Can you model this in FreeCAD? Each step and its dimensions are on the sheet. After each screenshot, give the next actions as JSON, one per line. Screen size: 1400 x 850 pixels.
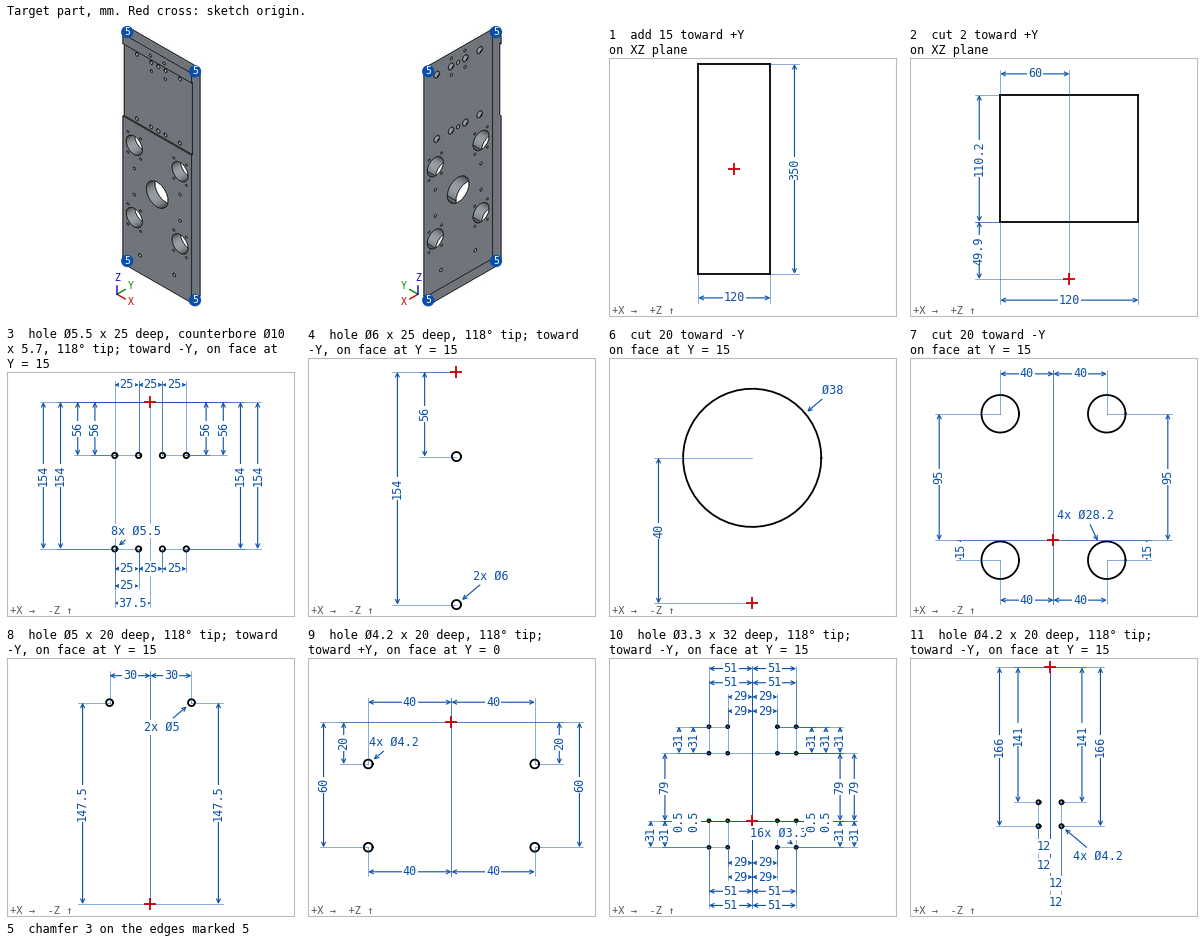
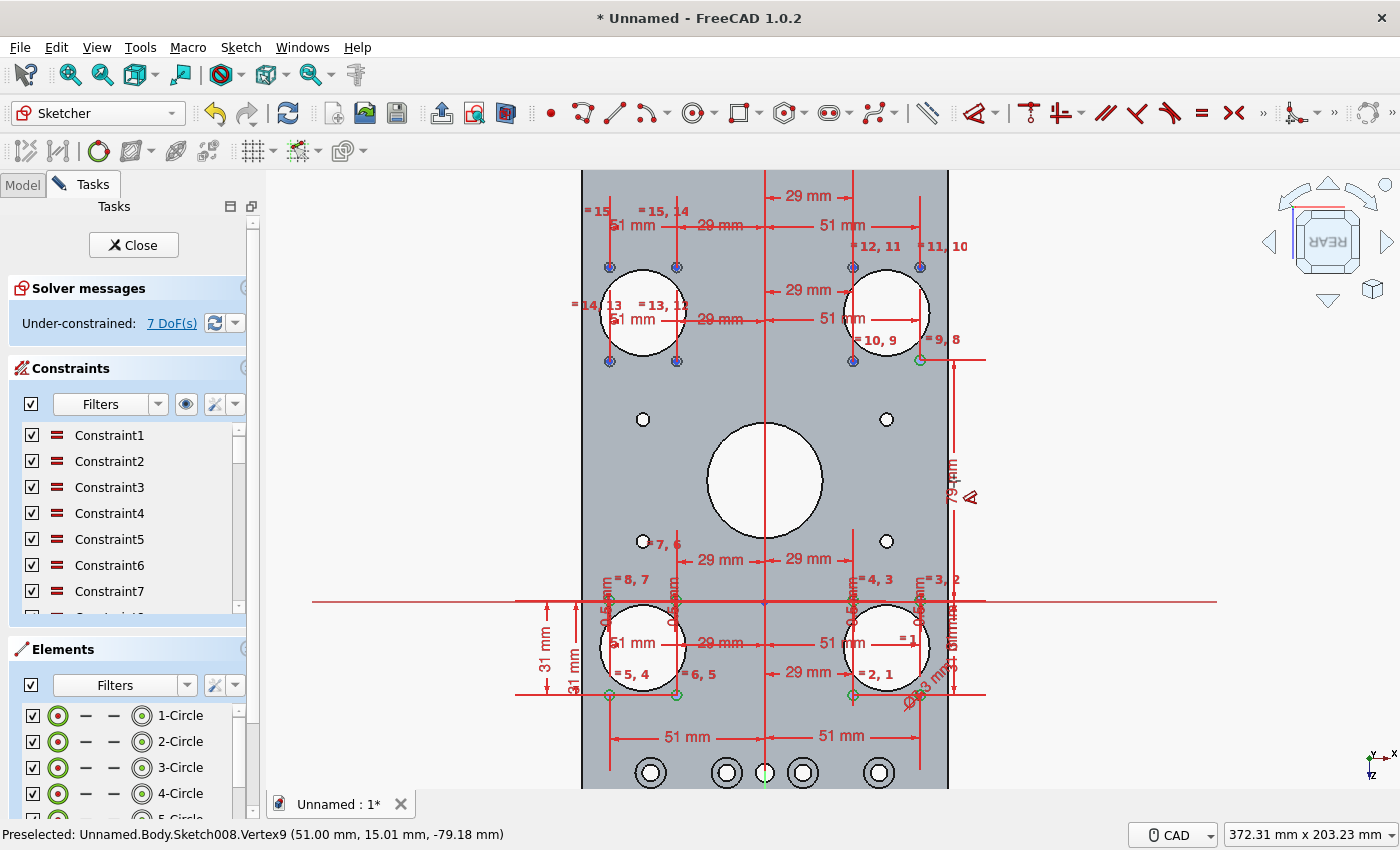
{"action": "left_click", "coordinate": [853, 601]}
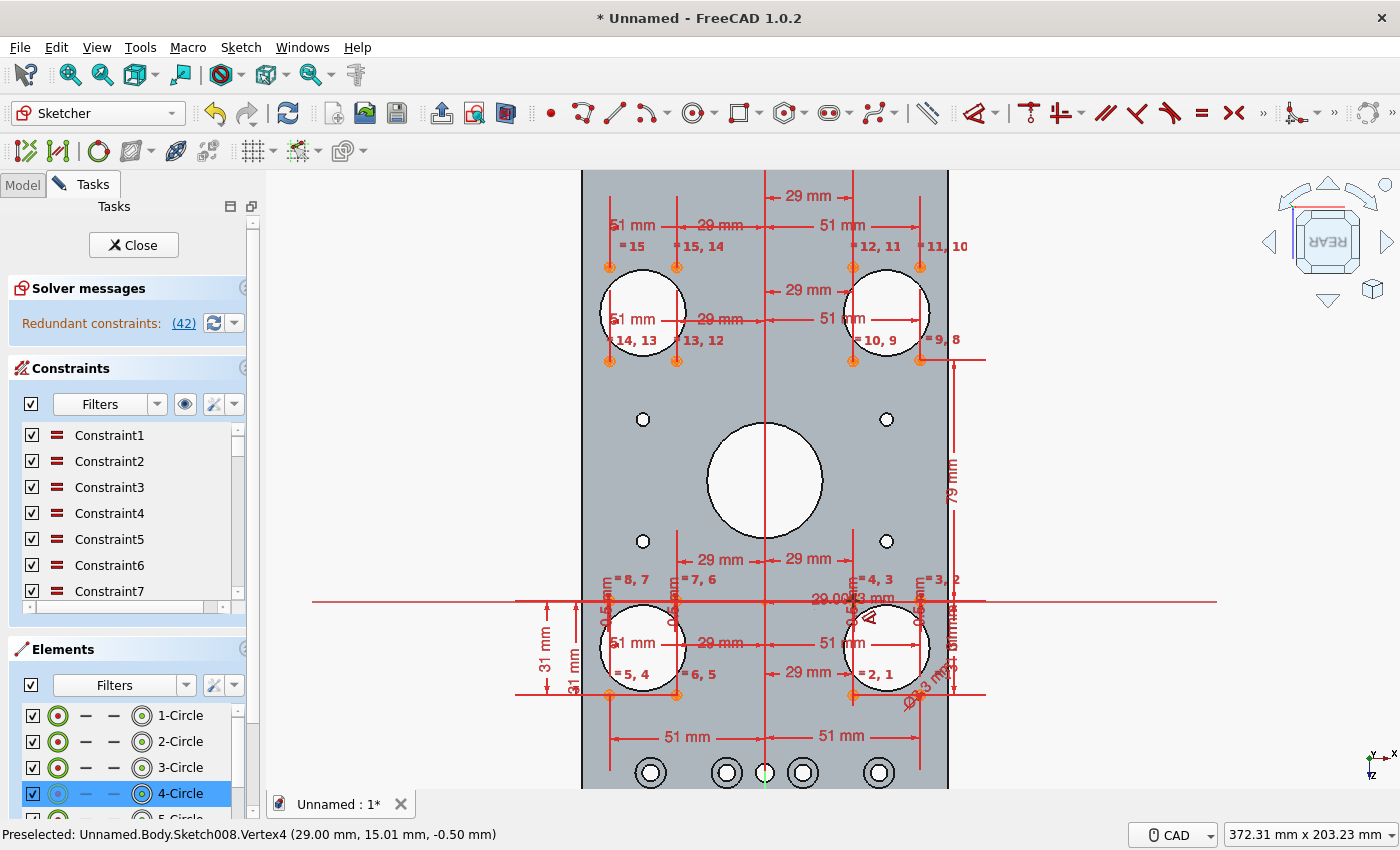
{"action": "left_click", "coordinate": [853, 361]}
{"action": "left_click", "coordinate": [887, 426]}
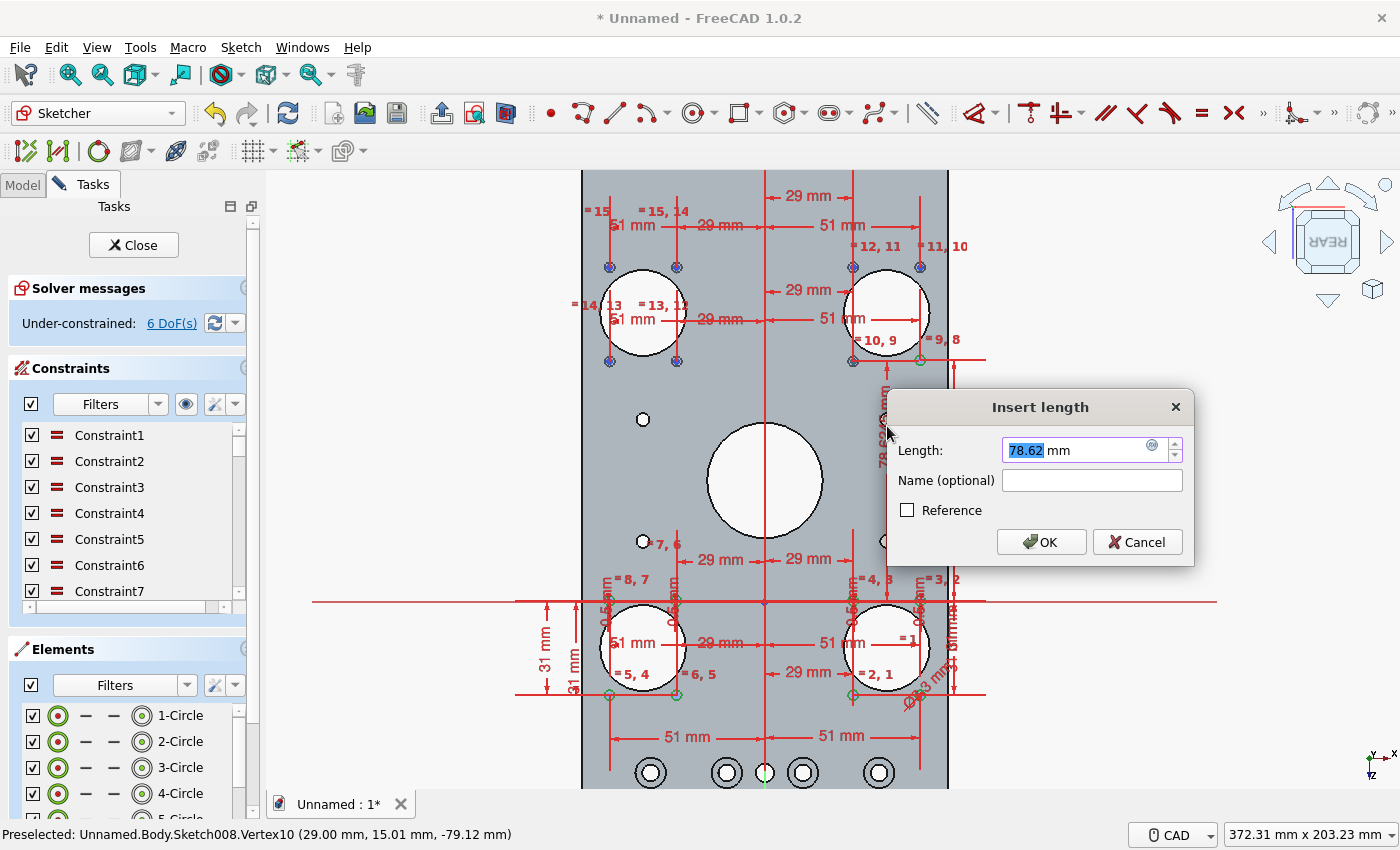
{"action": "type", "text": "79"}
{"action": "key", "text": "Return"}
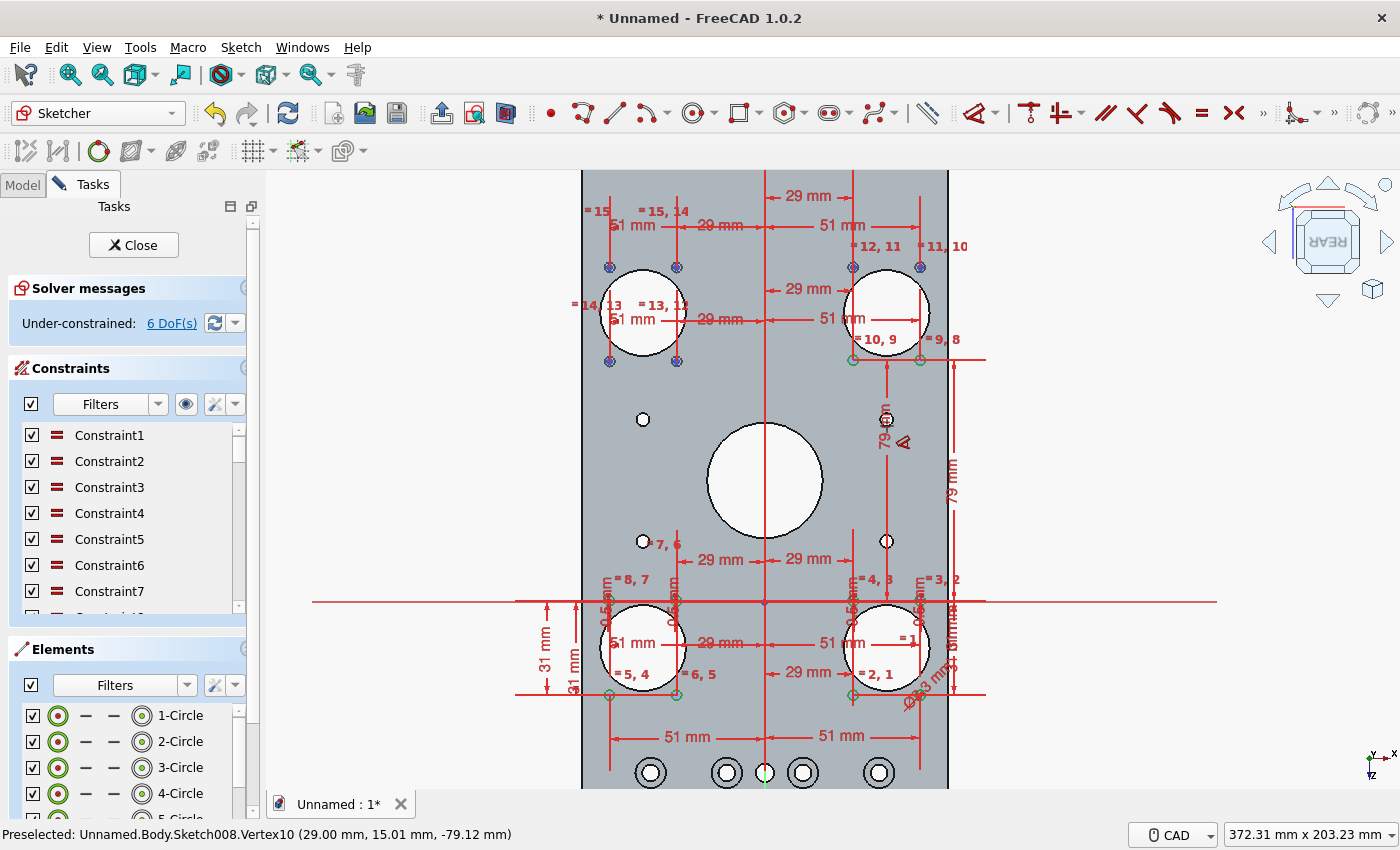
{"action": "left_click", "coordinate": [920, 360]}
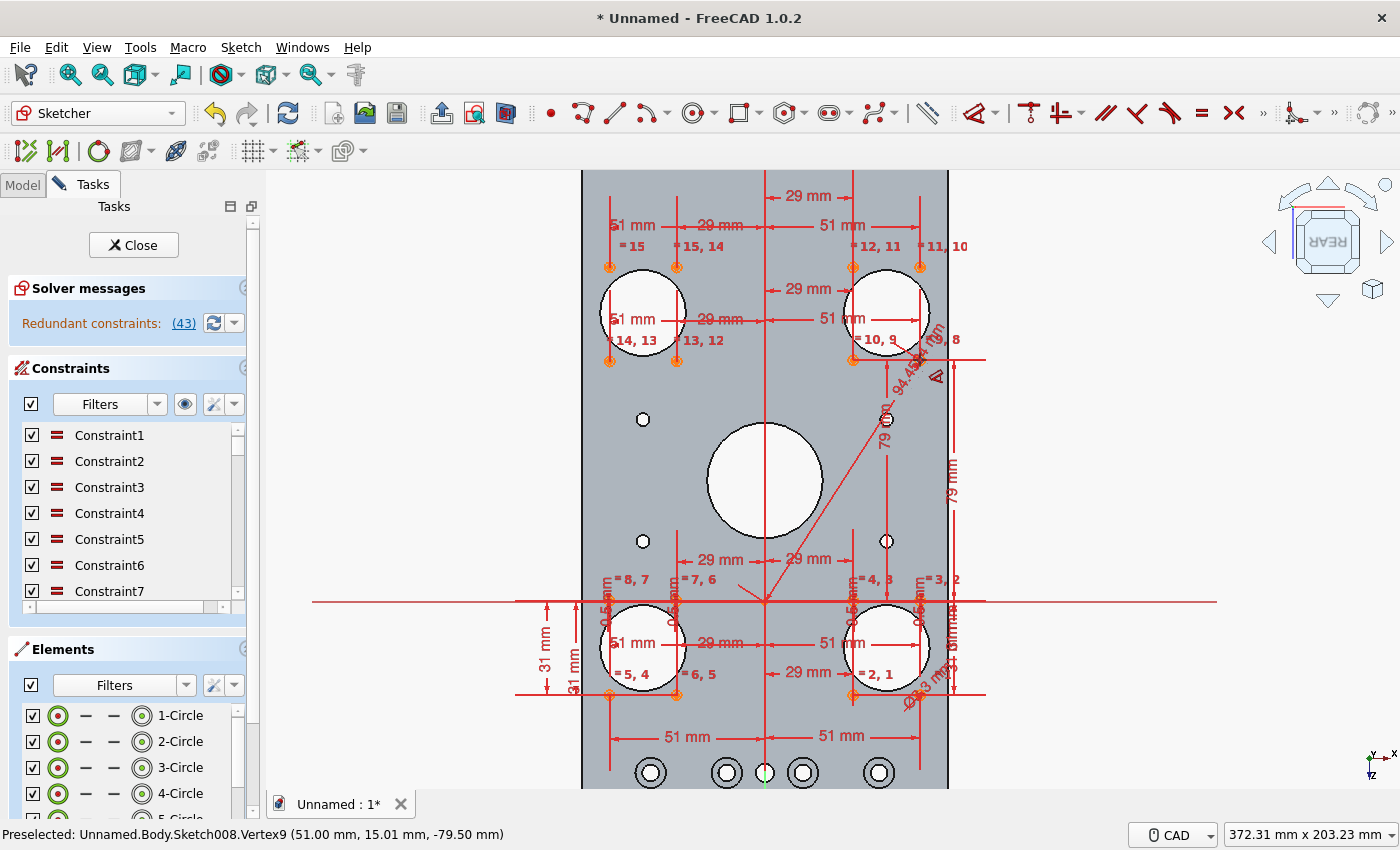
{"action": "left_click", "coordinate": [920, 267]}
{"action": "left_click", "coordinate": [954, 314]}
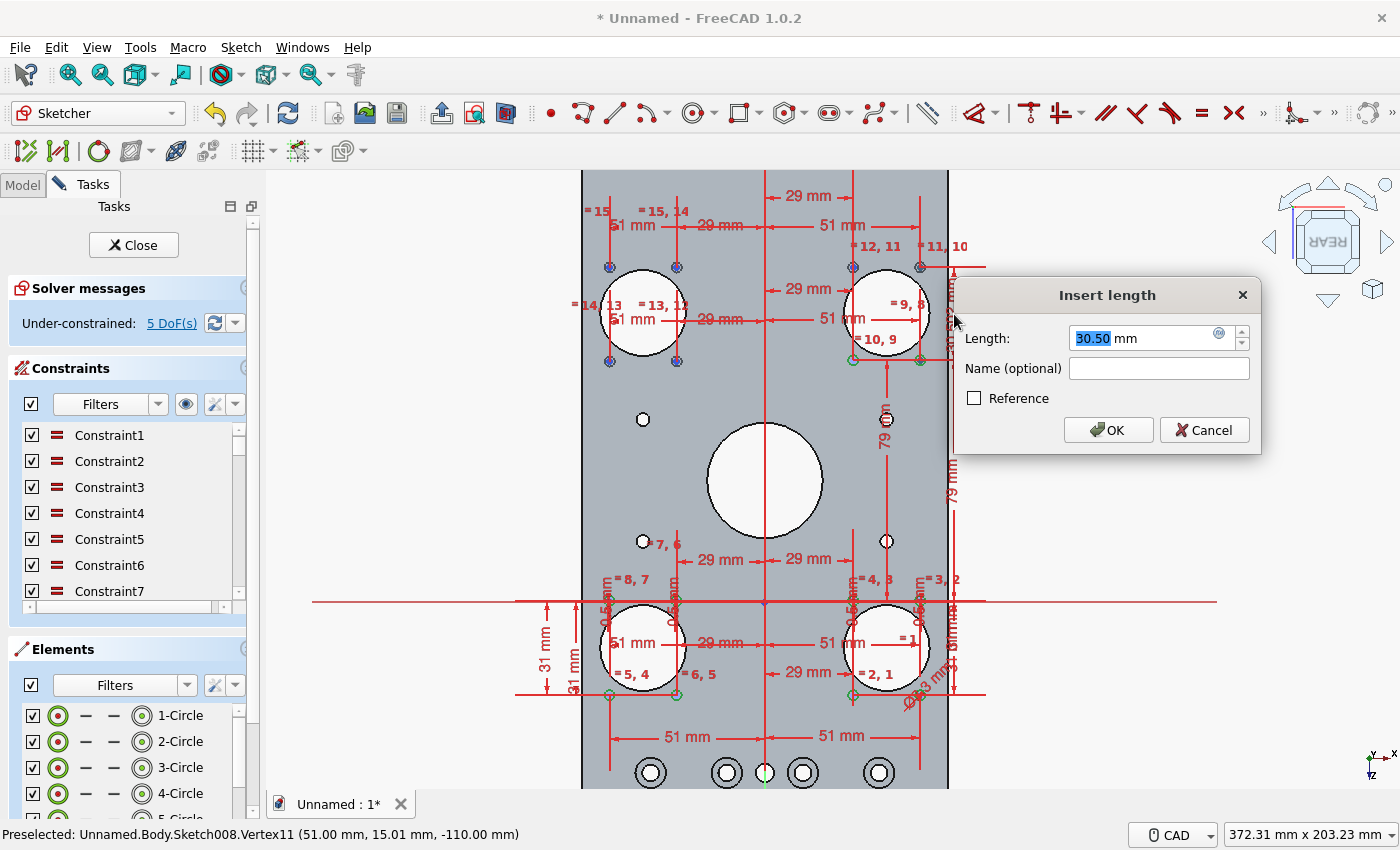
{"action": "type", "text": "31"}
{"action": "key", "text": "Return"}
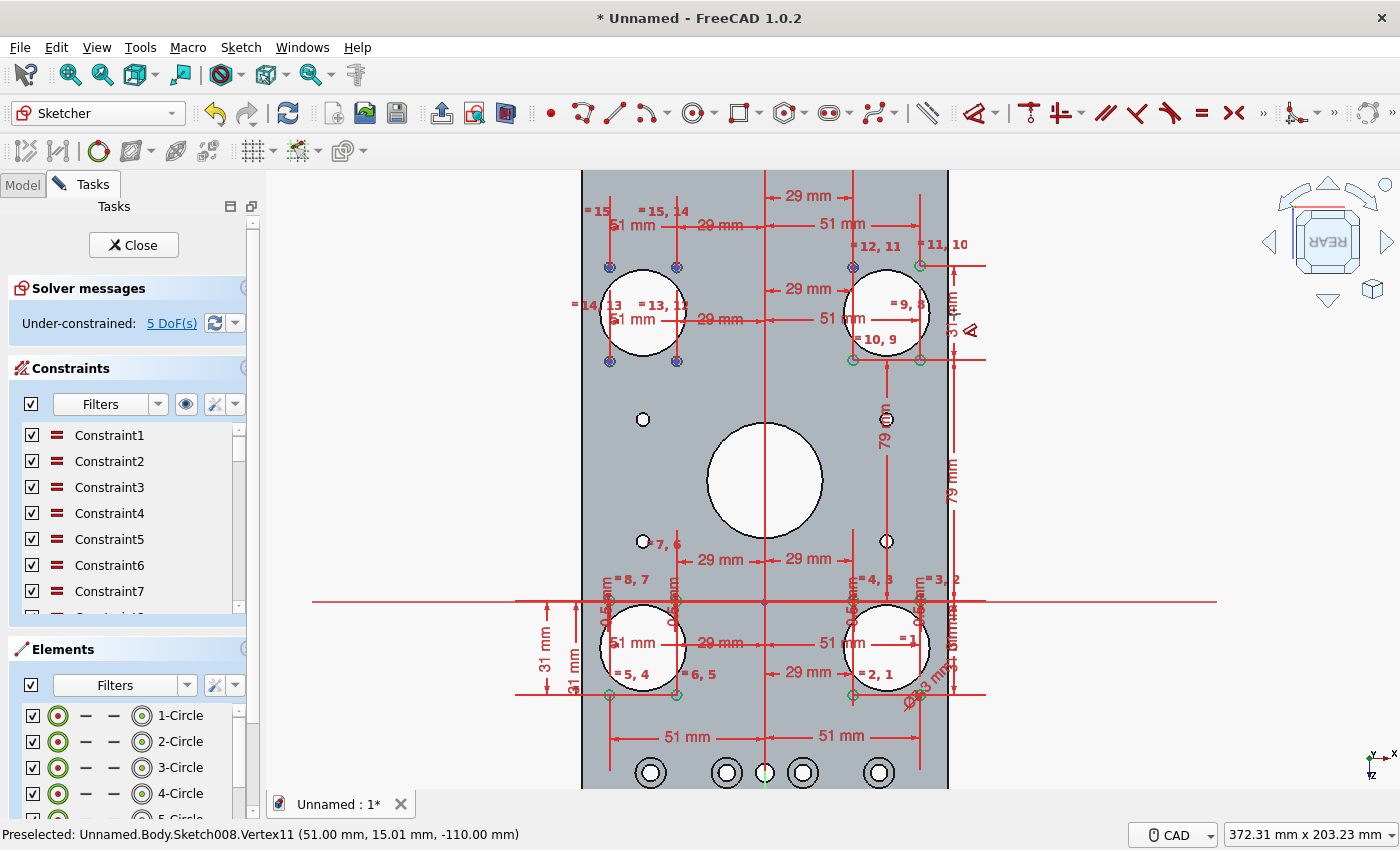
{"action": "left_click", "coordinate": [853, 360]}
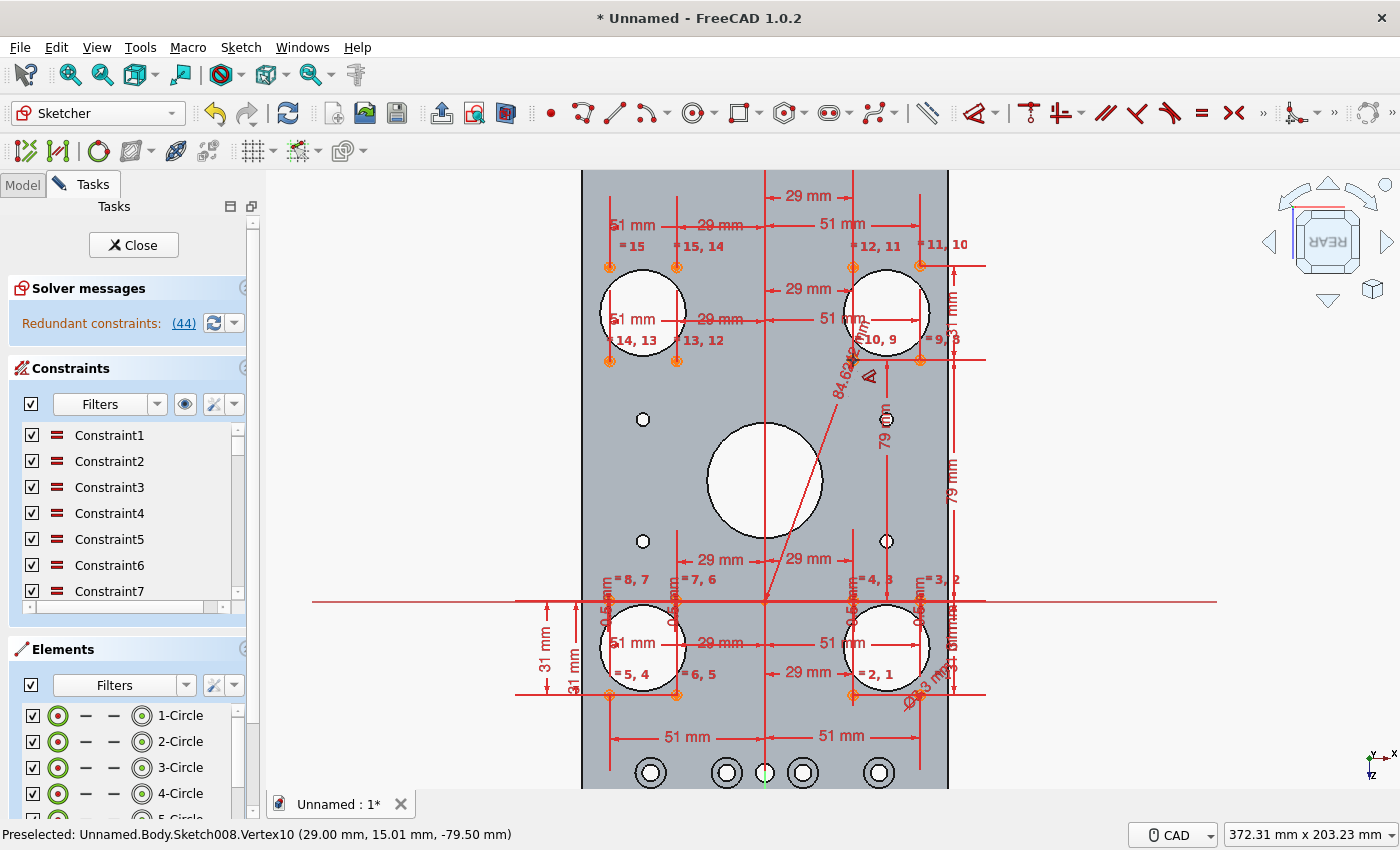
{"action": "left_click", "coordinate": [853, 267]}
{"action": "left_click", "coordinate": [887, 292]}